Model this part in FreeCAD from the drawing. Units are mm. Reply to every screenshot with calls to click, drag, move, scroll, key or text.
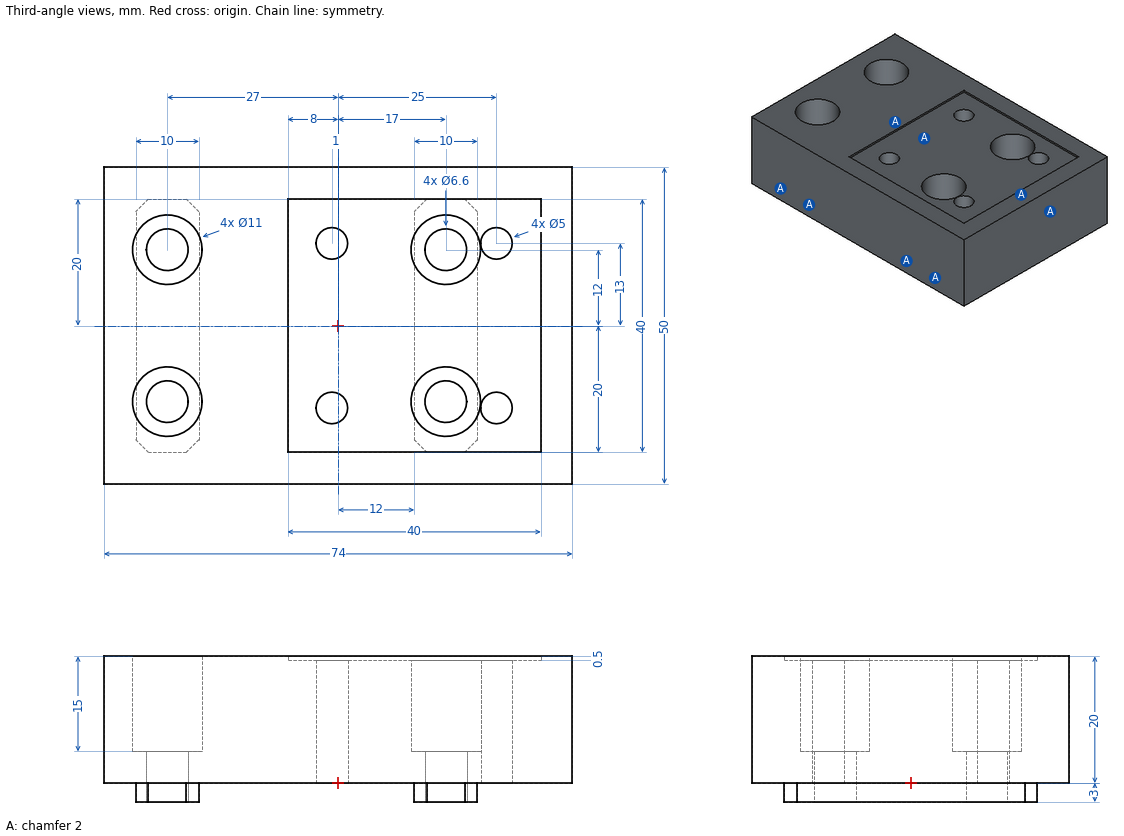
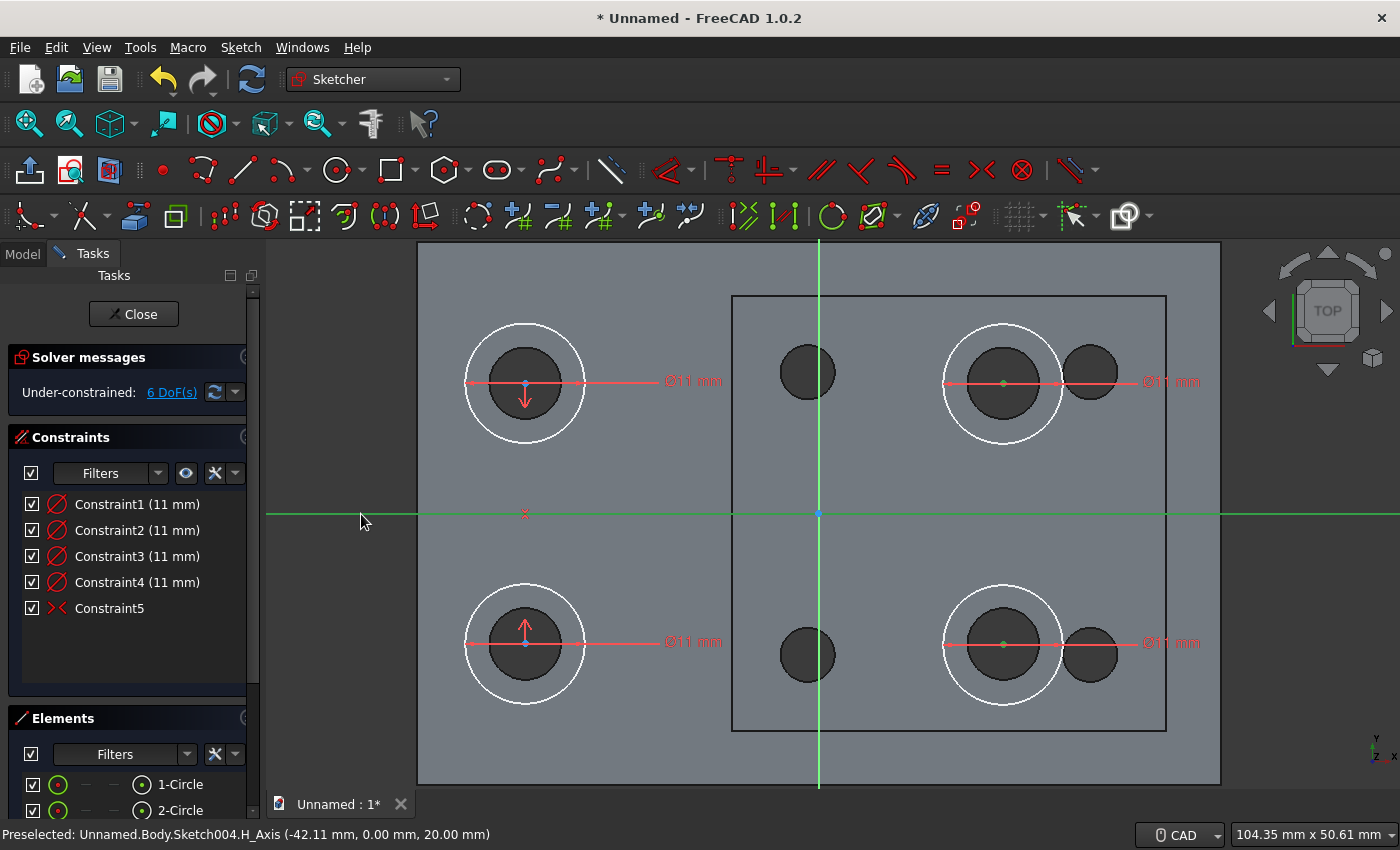
click(982, 170)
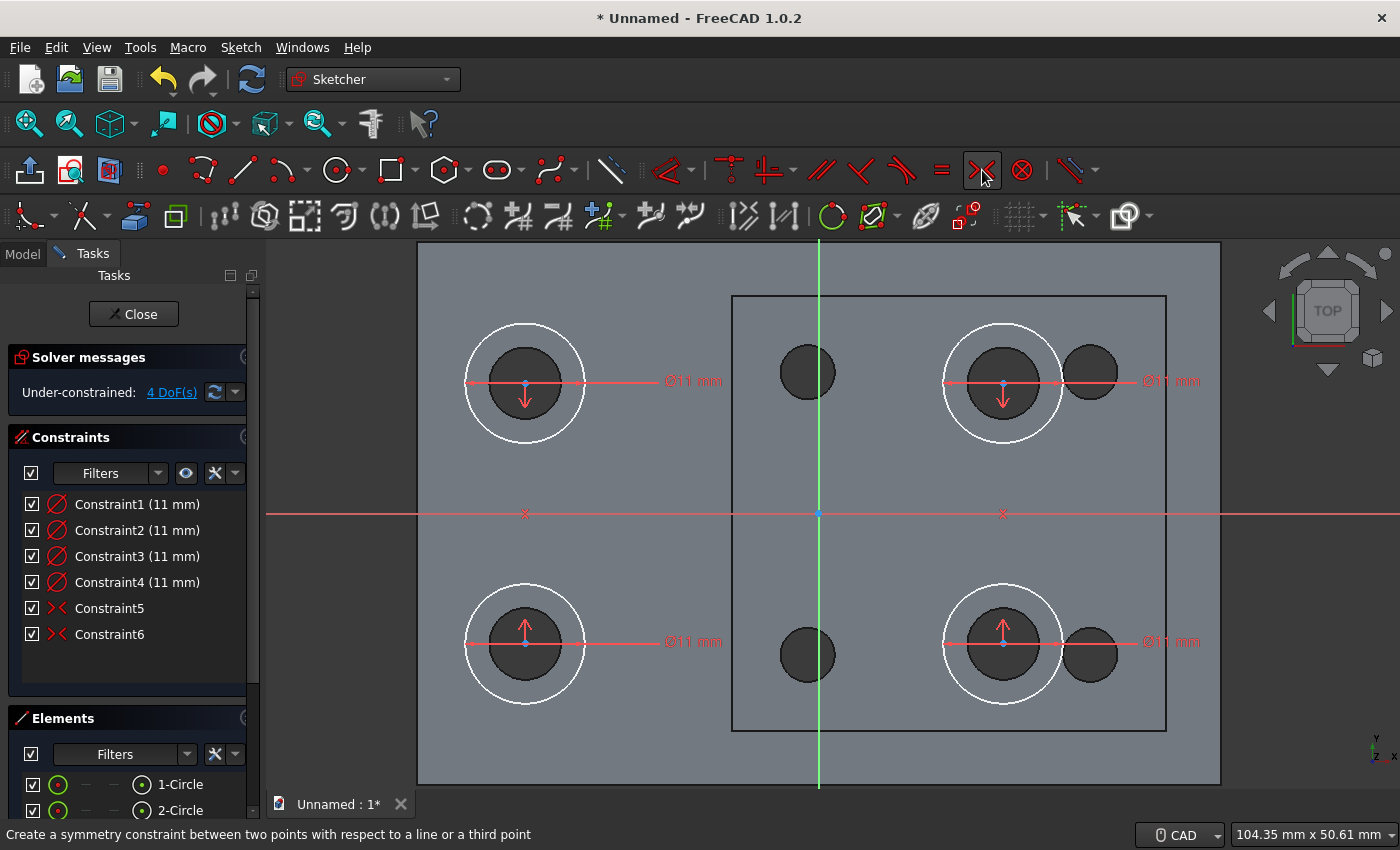
click(666, 170)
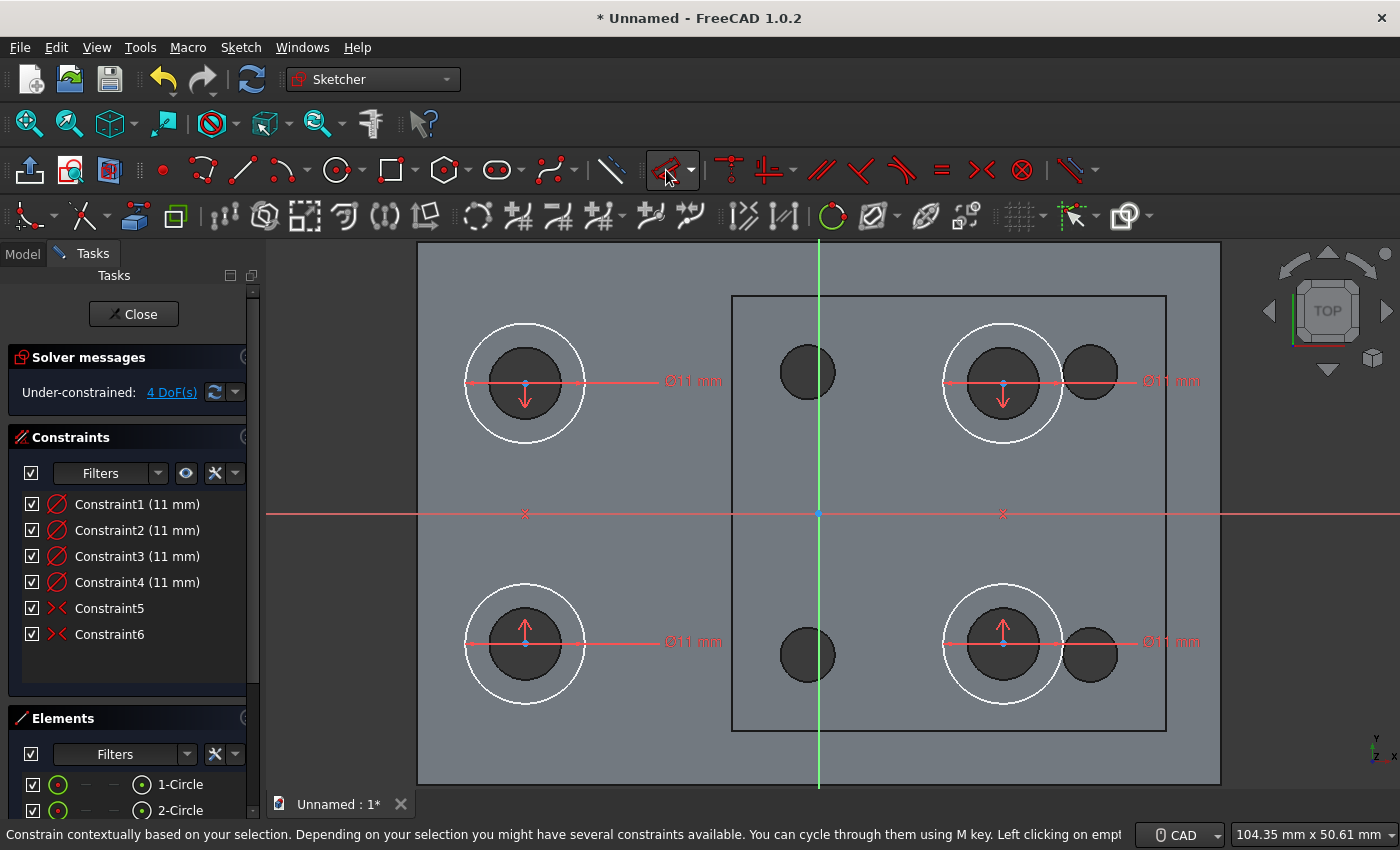
click(525, 383)
click(672, 349)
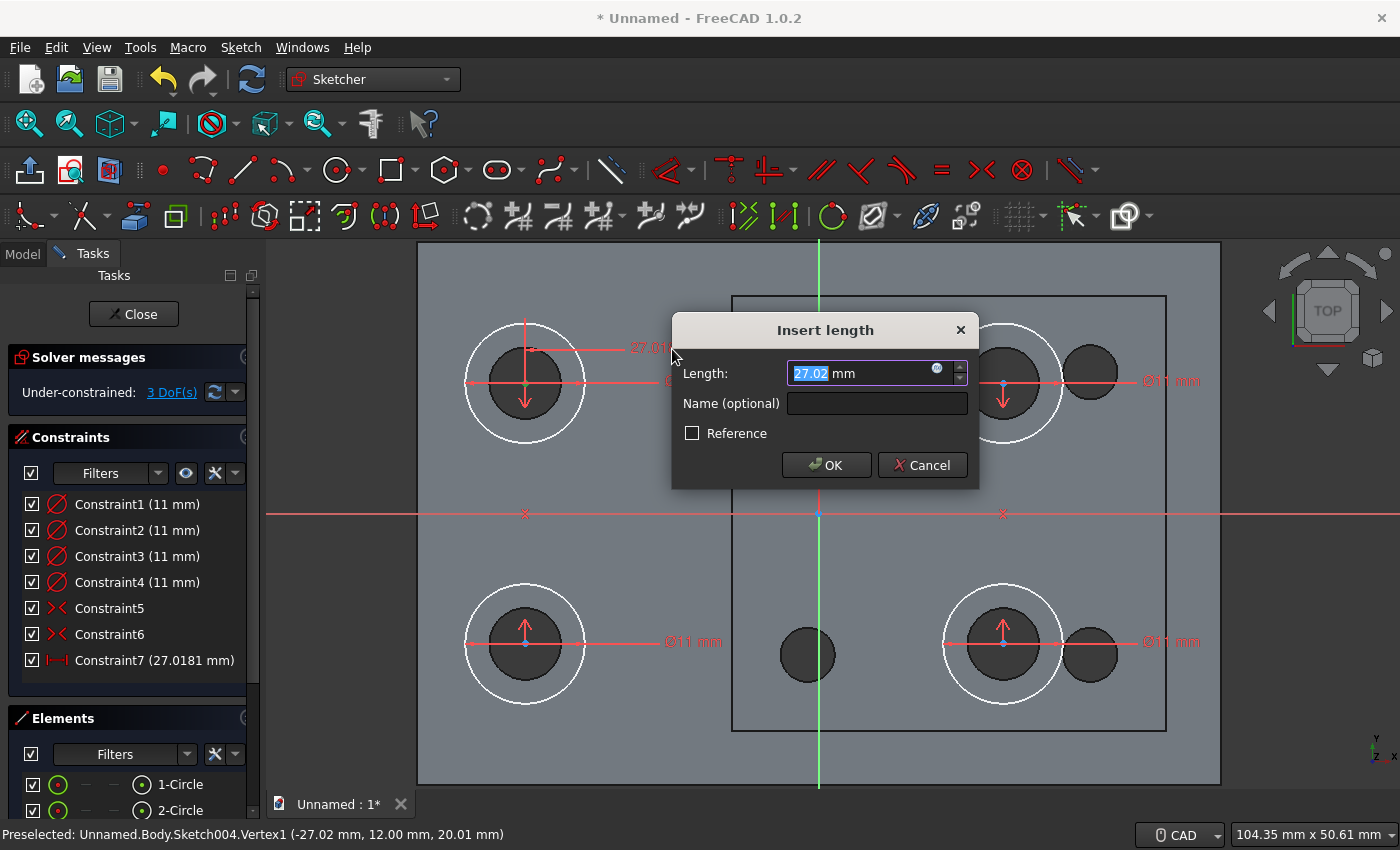
text(27)
key(Return)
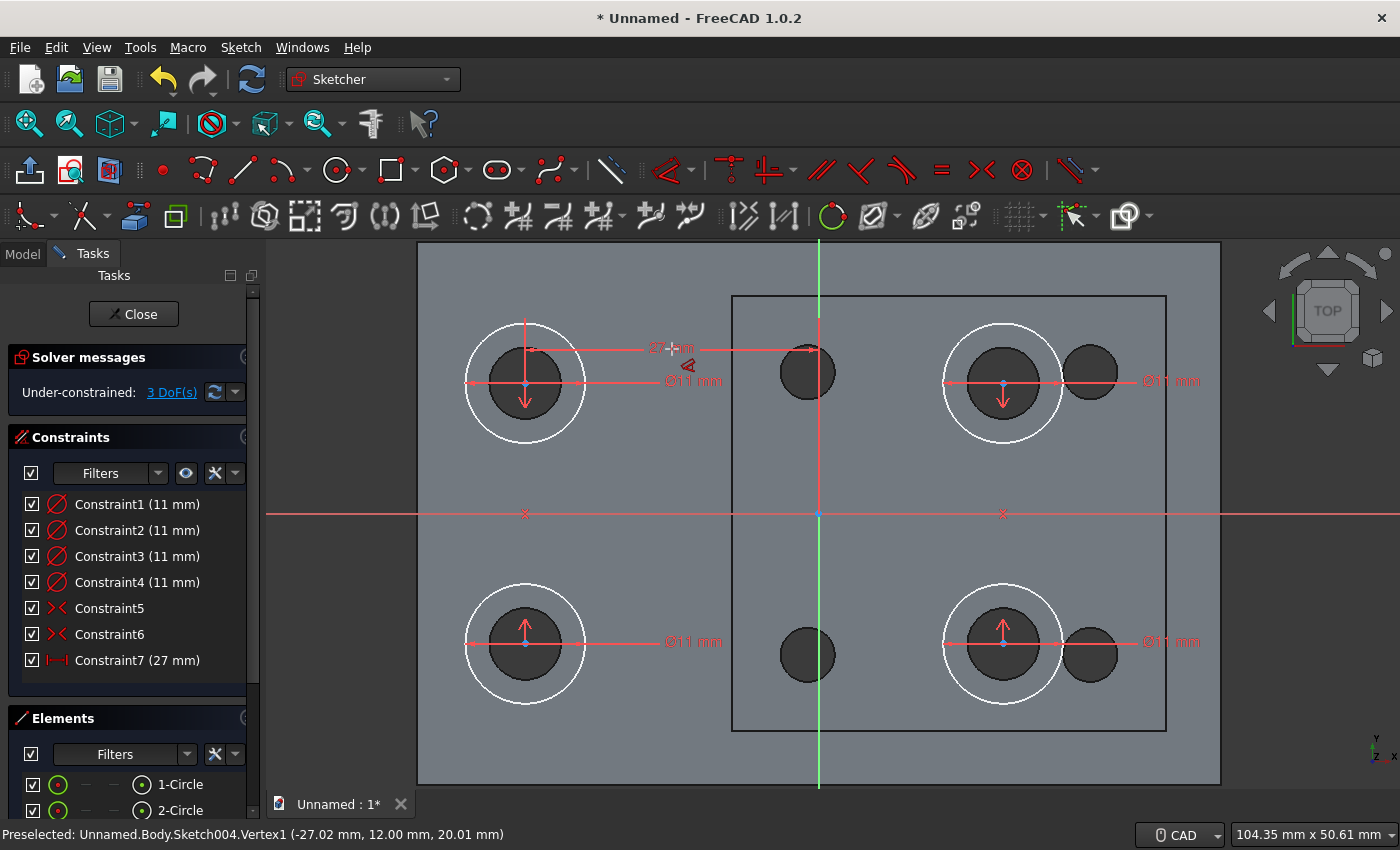
click(525, 383)
click(491, 448)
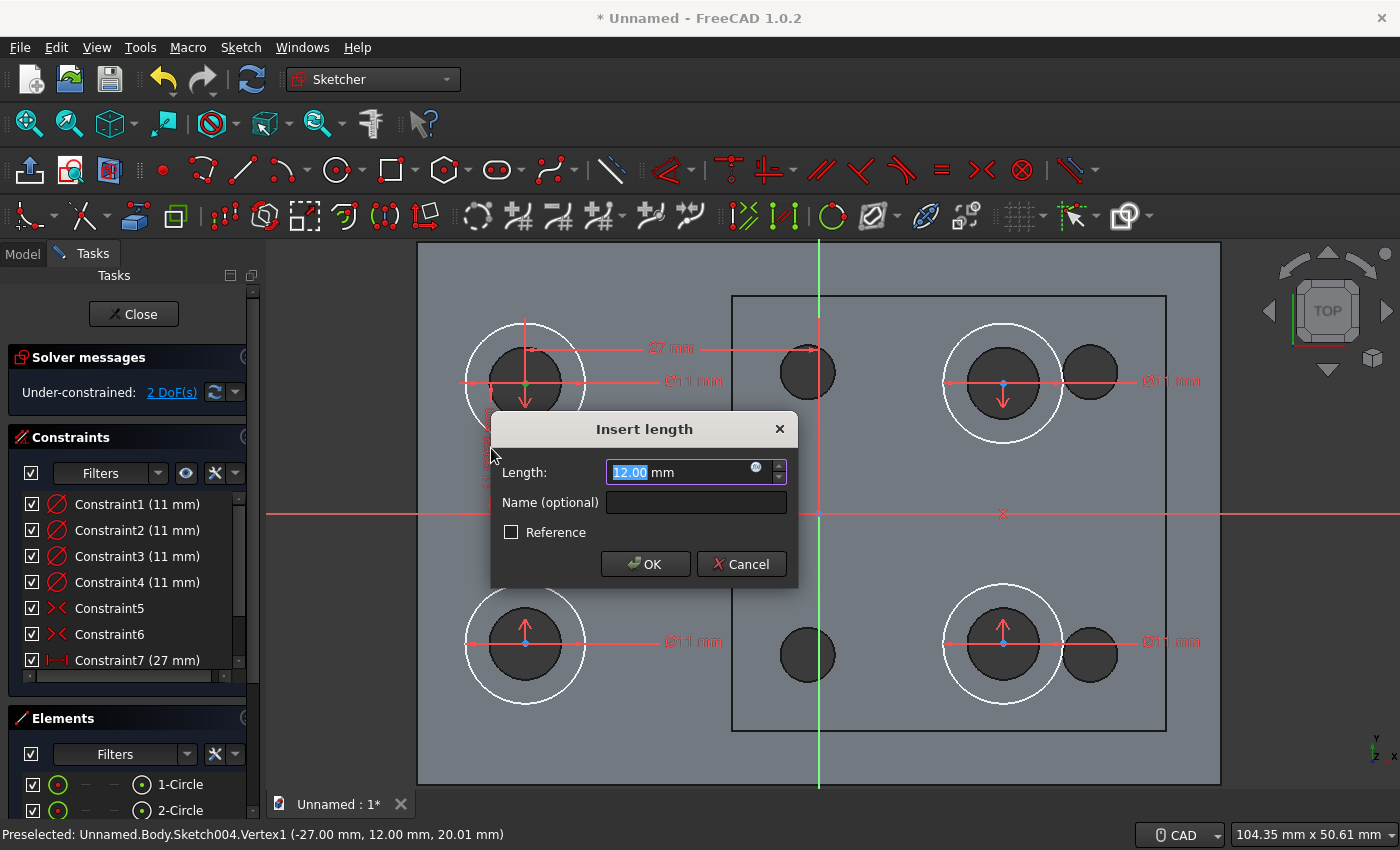
text(12)
key(Return)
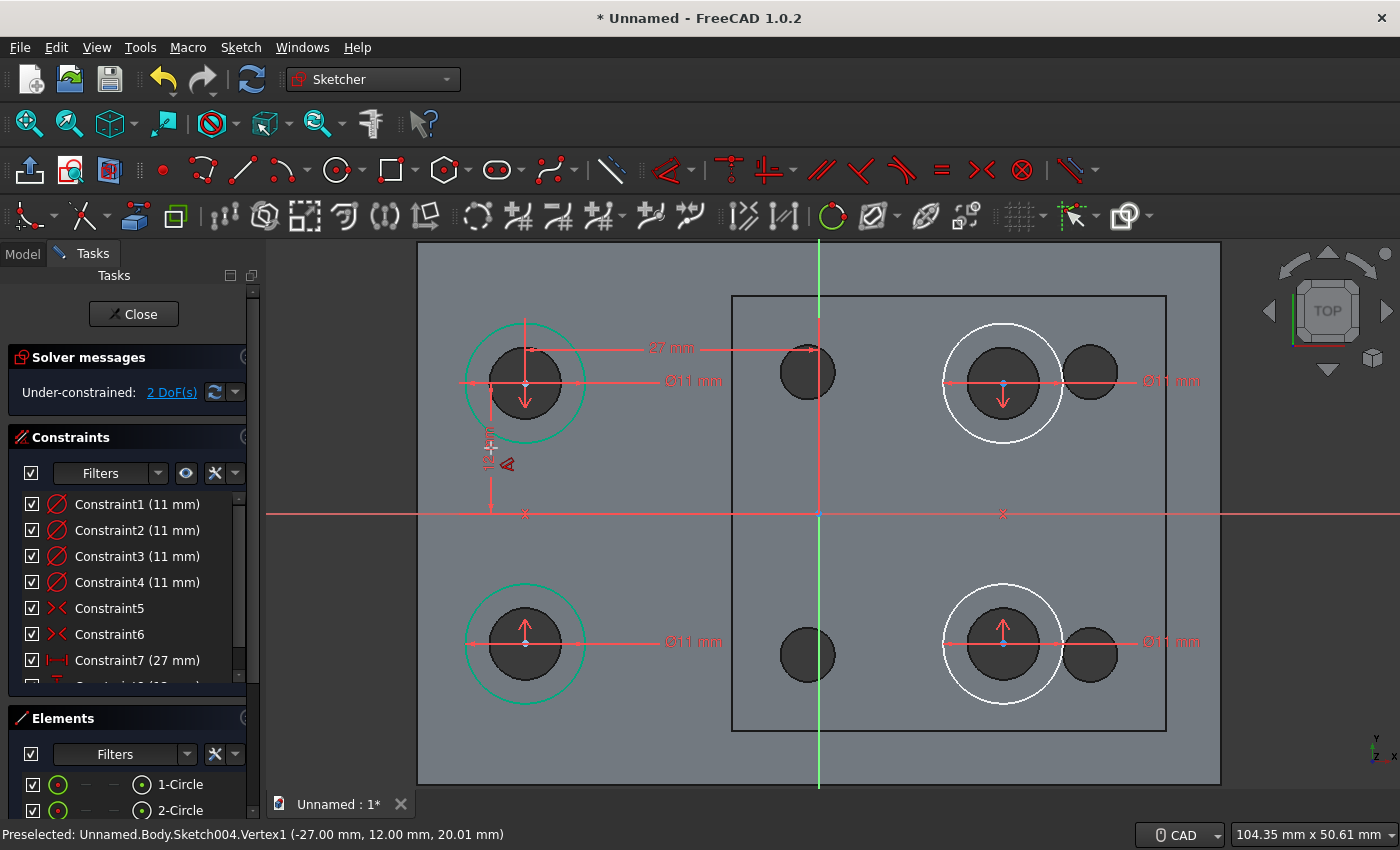
click(1003, 383)
click(911, 349)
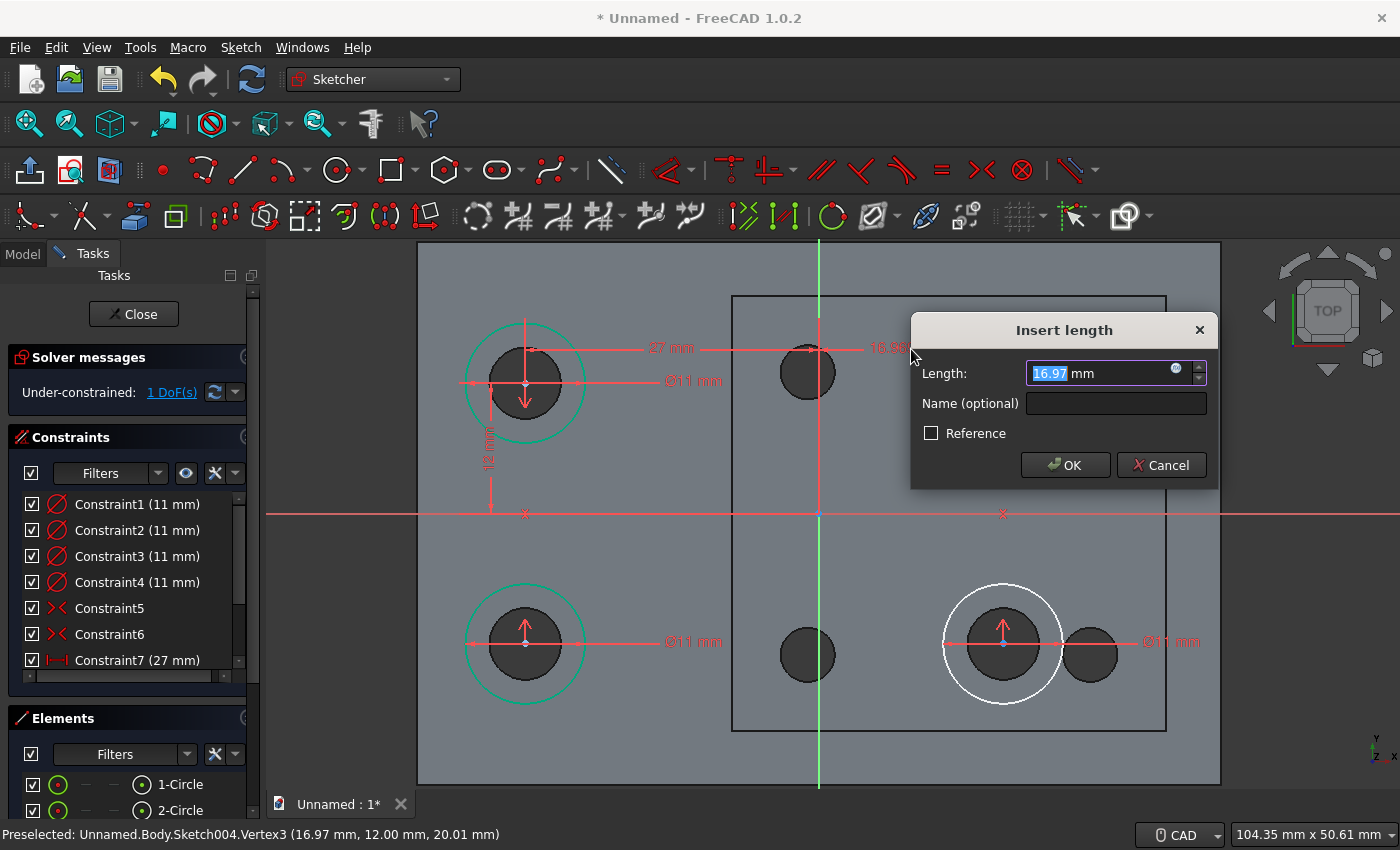
text(17)
key(Return)